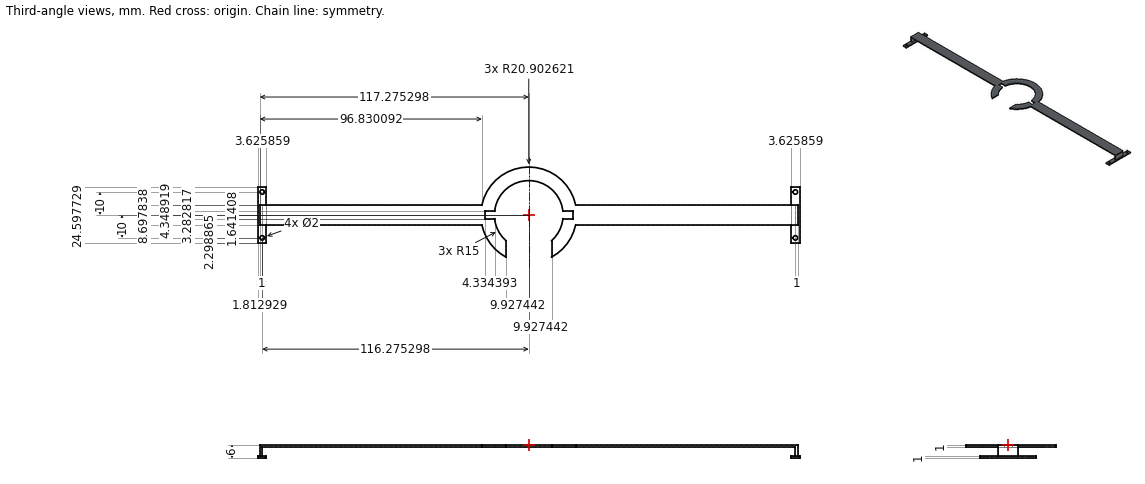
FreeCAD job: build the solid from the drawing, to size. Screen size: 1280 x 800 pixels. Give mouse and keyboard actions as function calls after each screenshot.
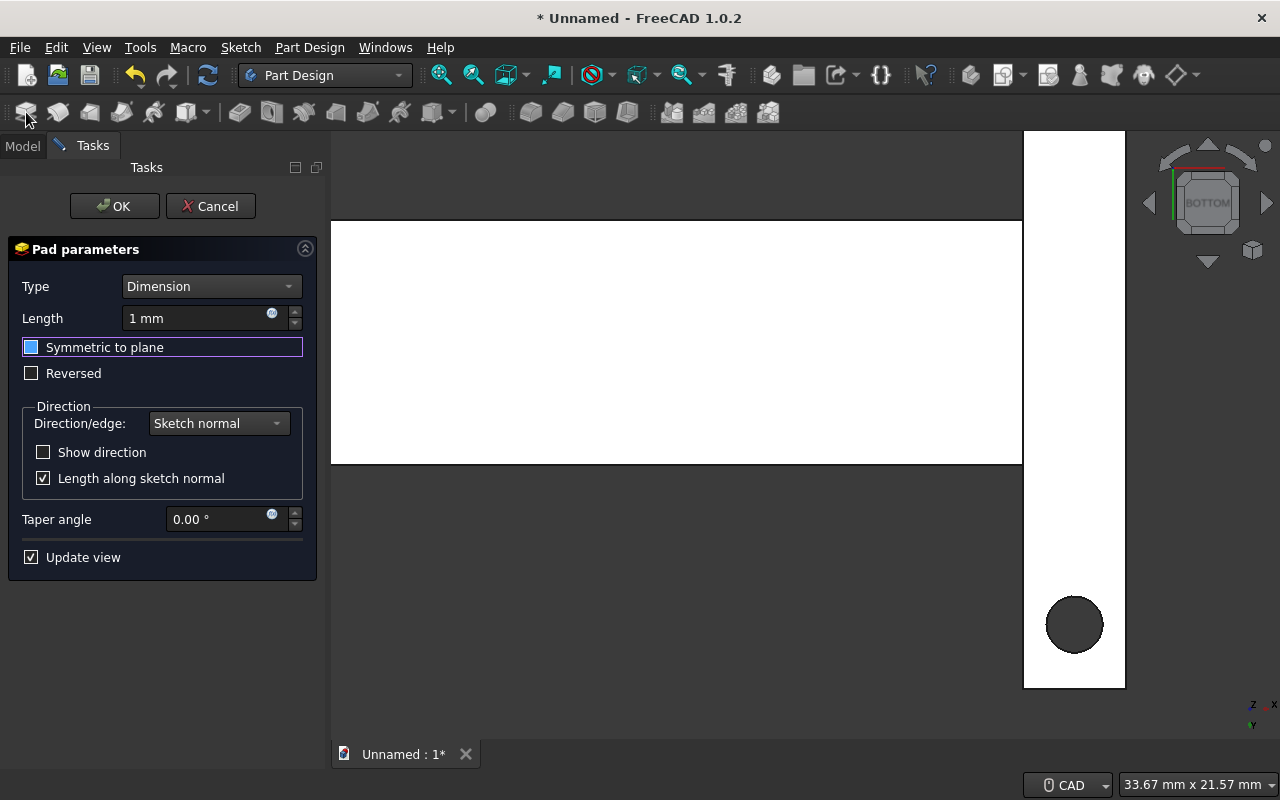
click(30, 373)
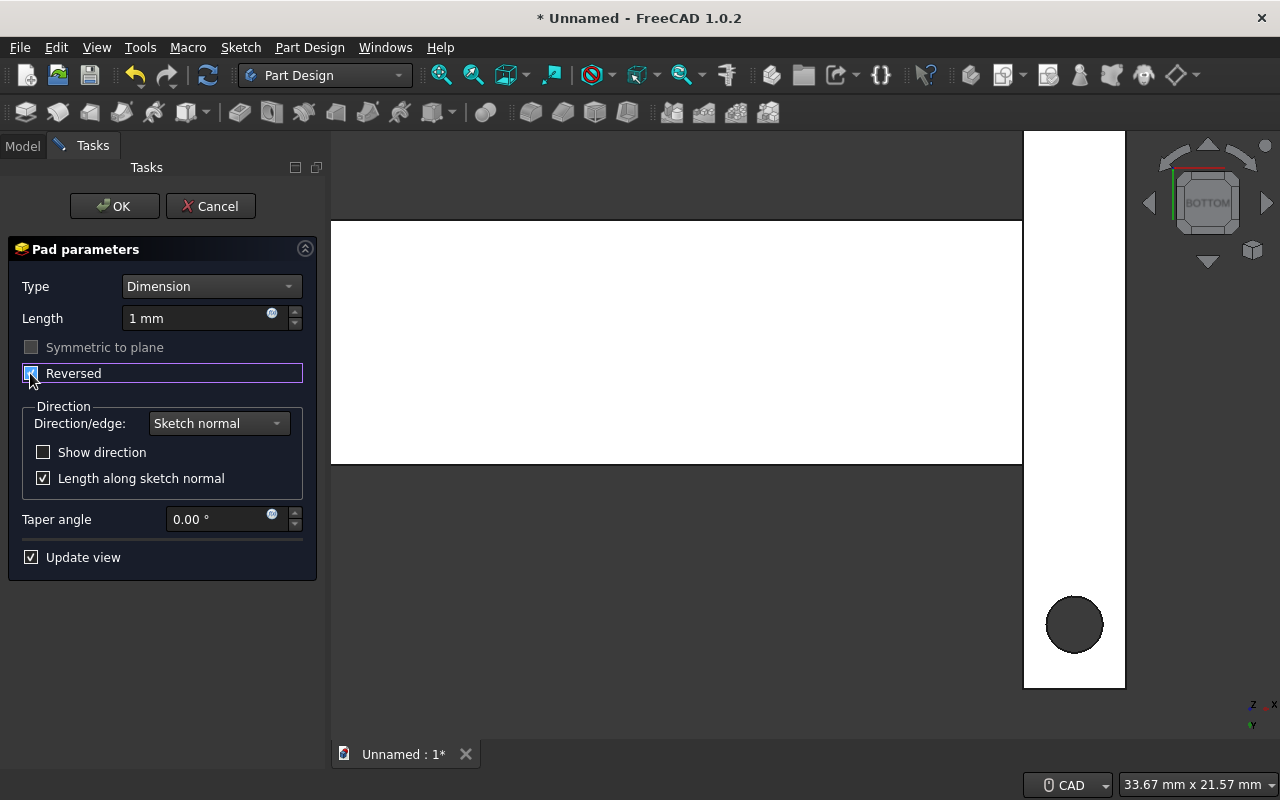
click(115, 206)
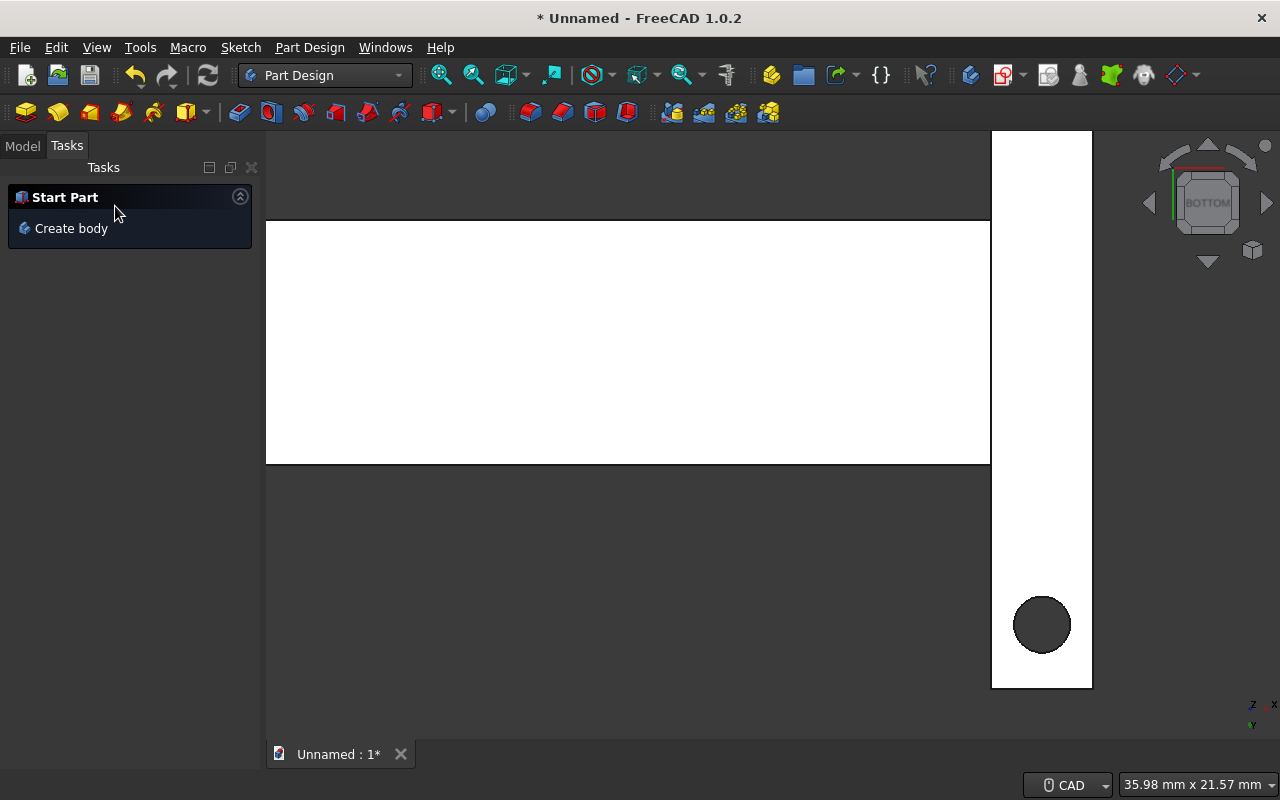
key(0)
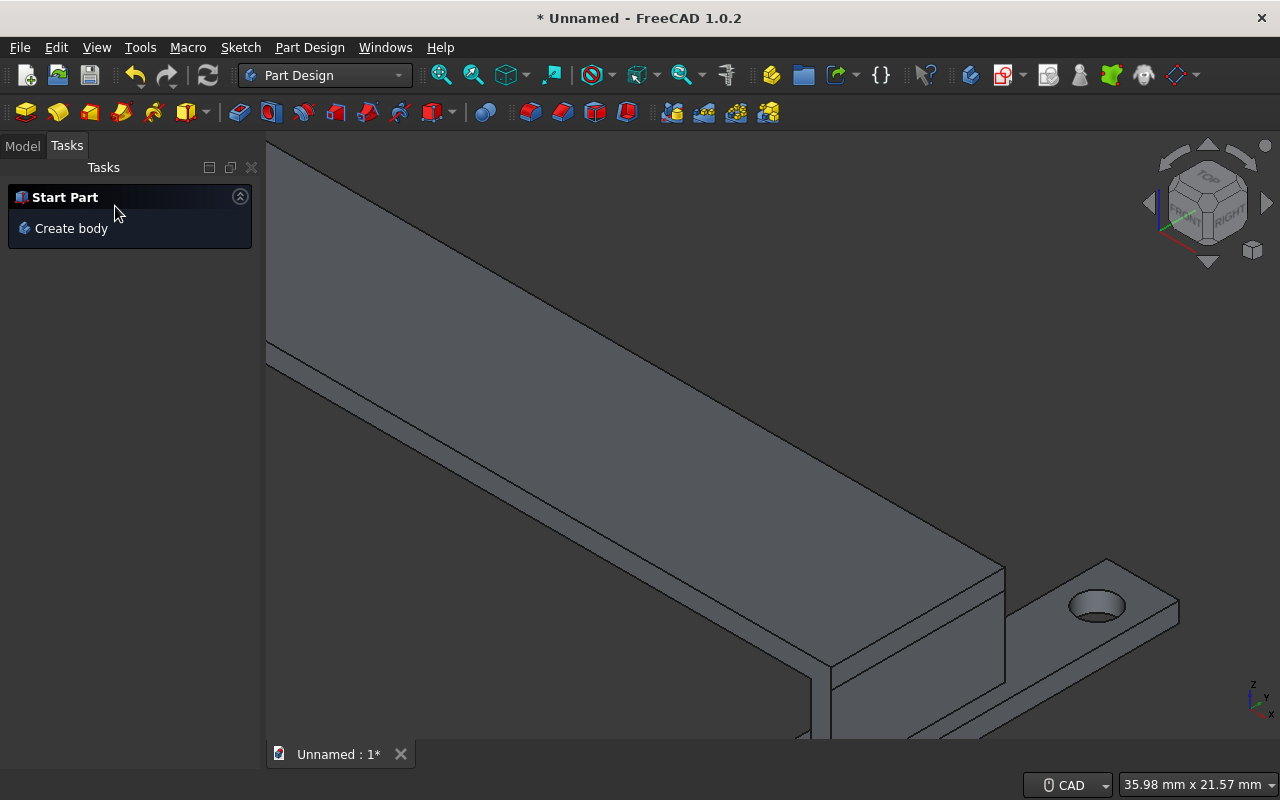
click(442, 76)